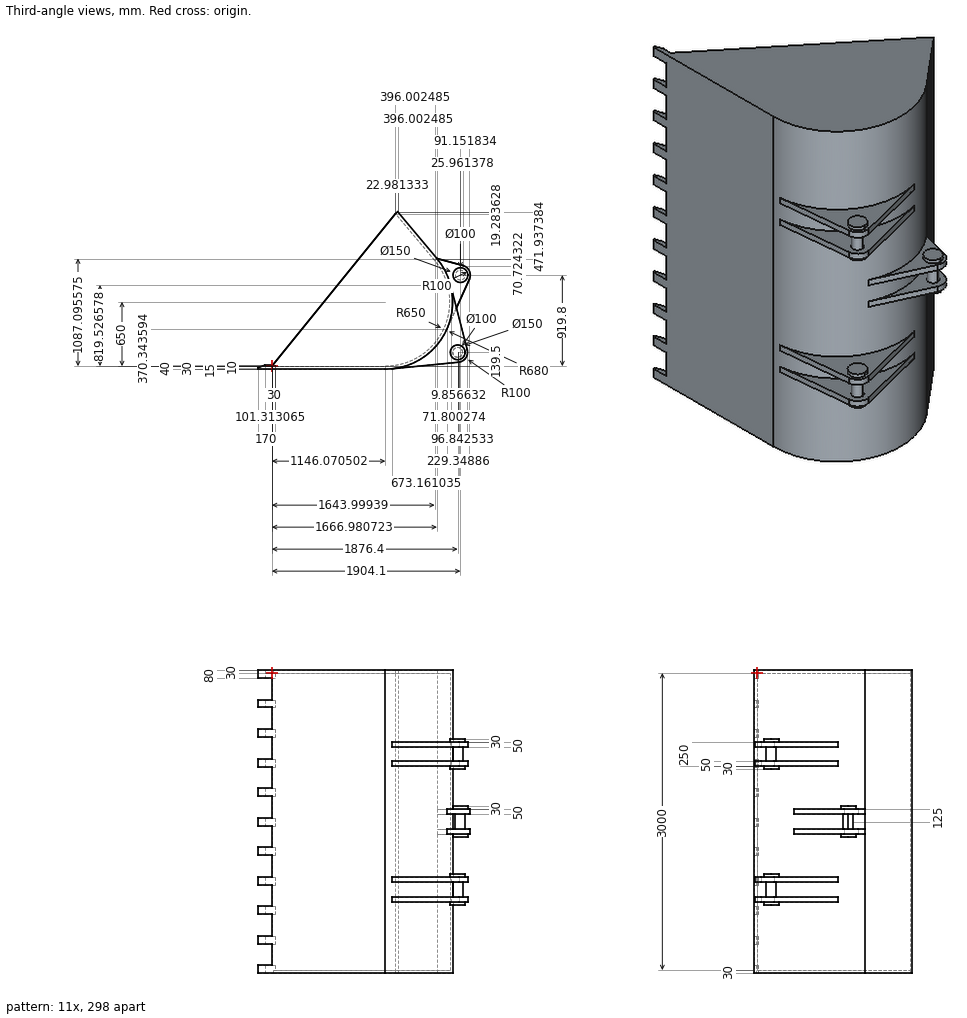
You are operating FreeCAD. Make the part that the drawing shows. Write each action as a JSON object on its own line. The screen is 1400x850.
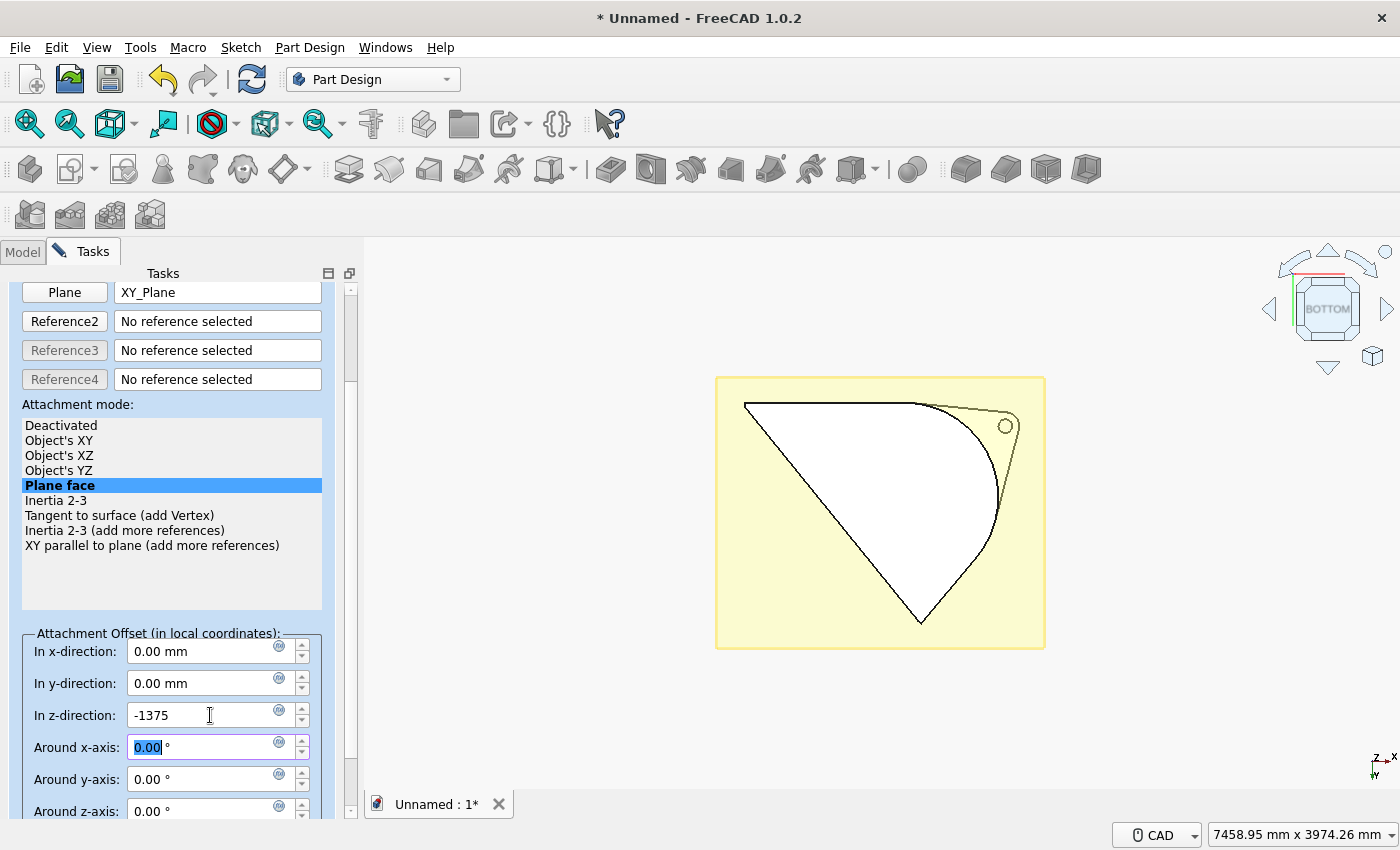
{"action": "scroll", "coordinate": [351, 550], "scroll_direction": "up", "scroll_amount": 3}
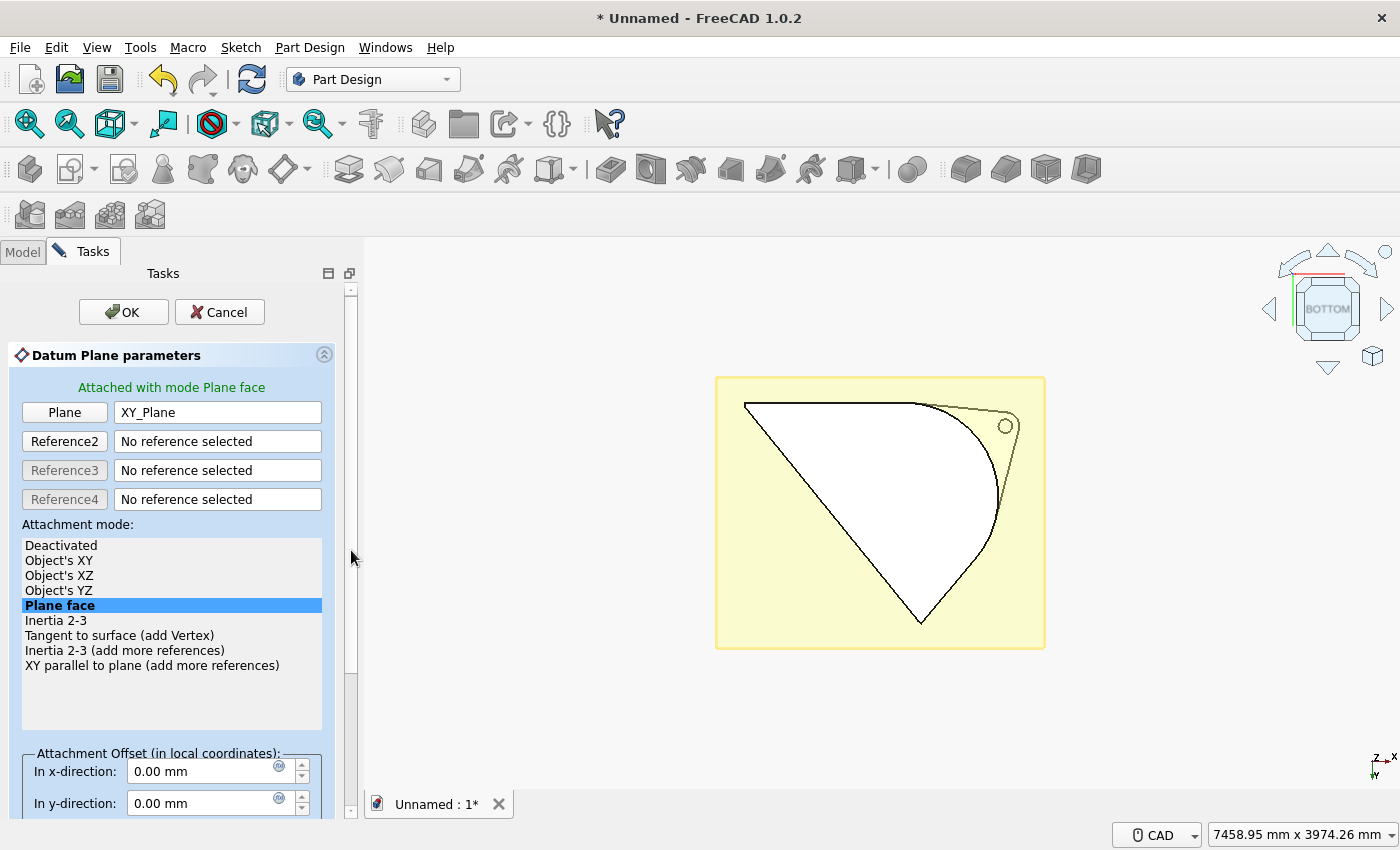
{"action": "left_click", "coordinate": [124, 312]}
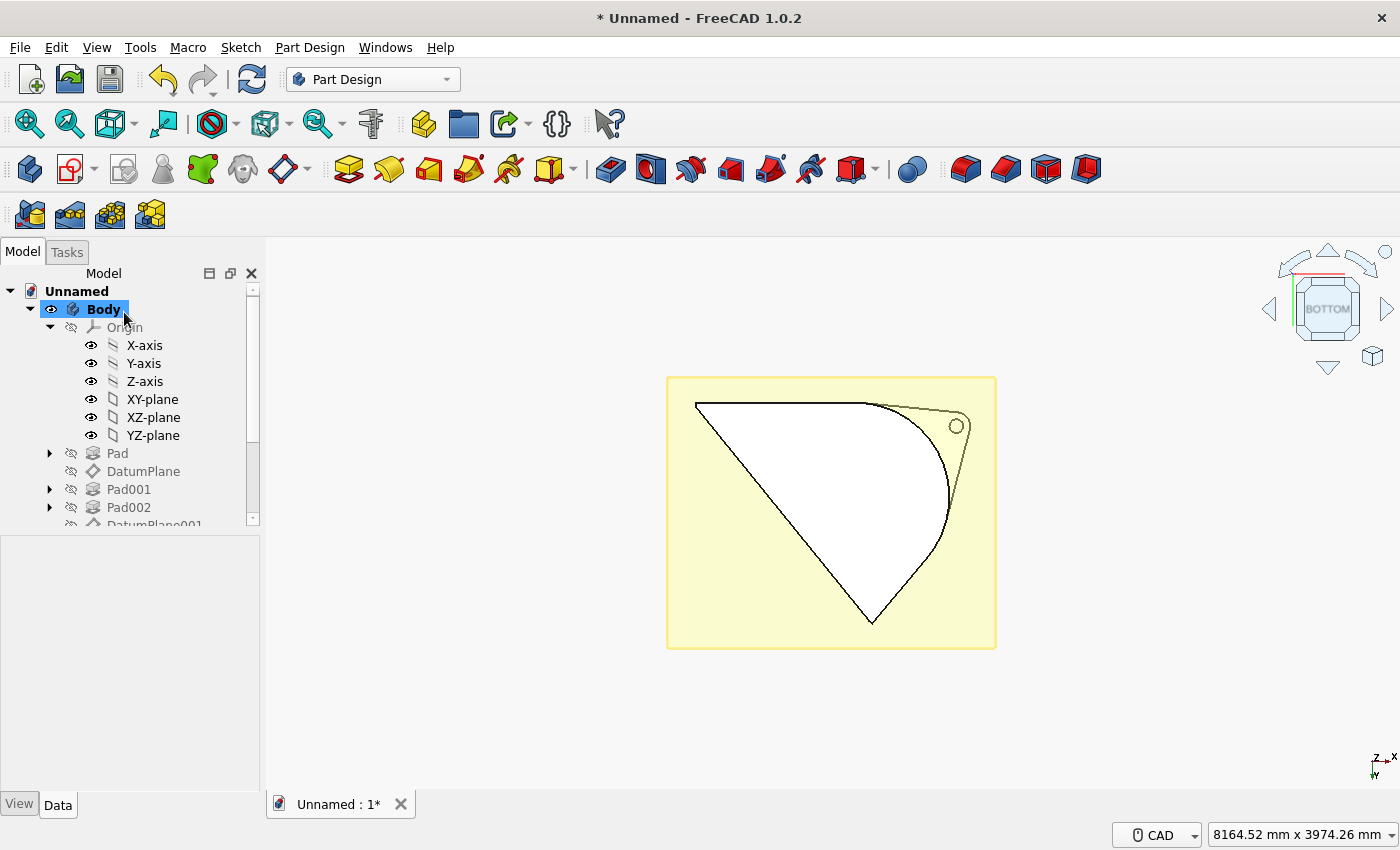
{"action": "scroll", "coordinate": [100, 413], "scroll_direction": "down", "scroll_amount": 3}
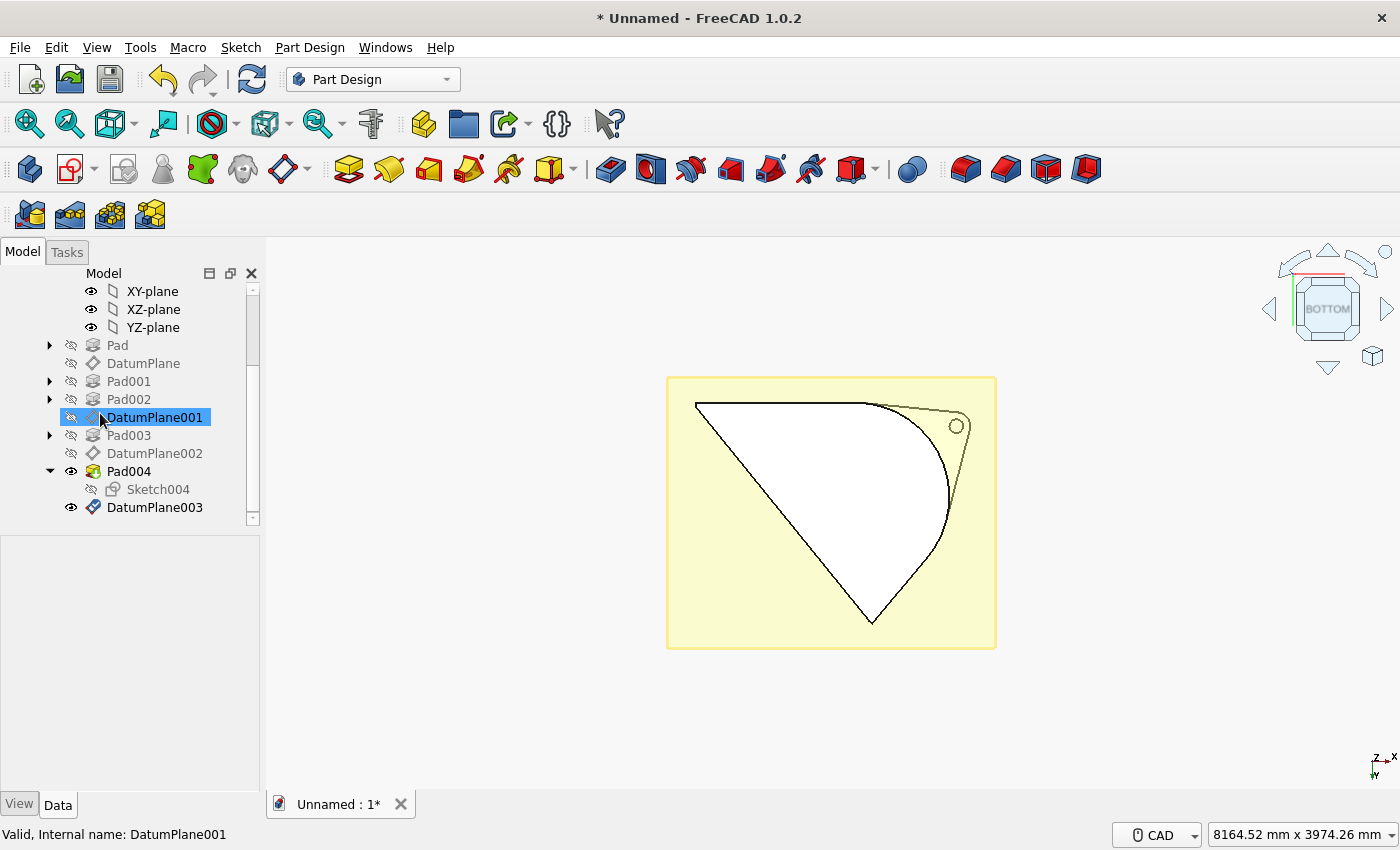
{"action": "left_click", "coordinate": [116, 507]}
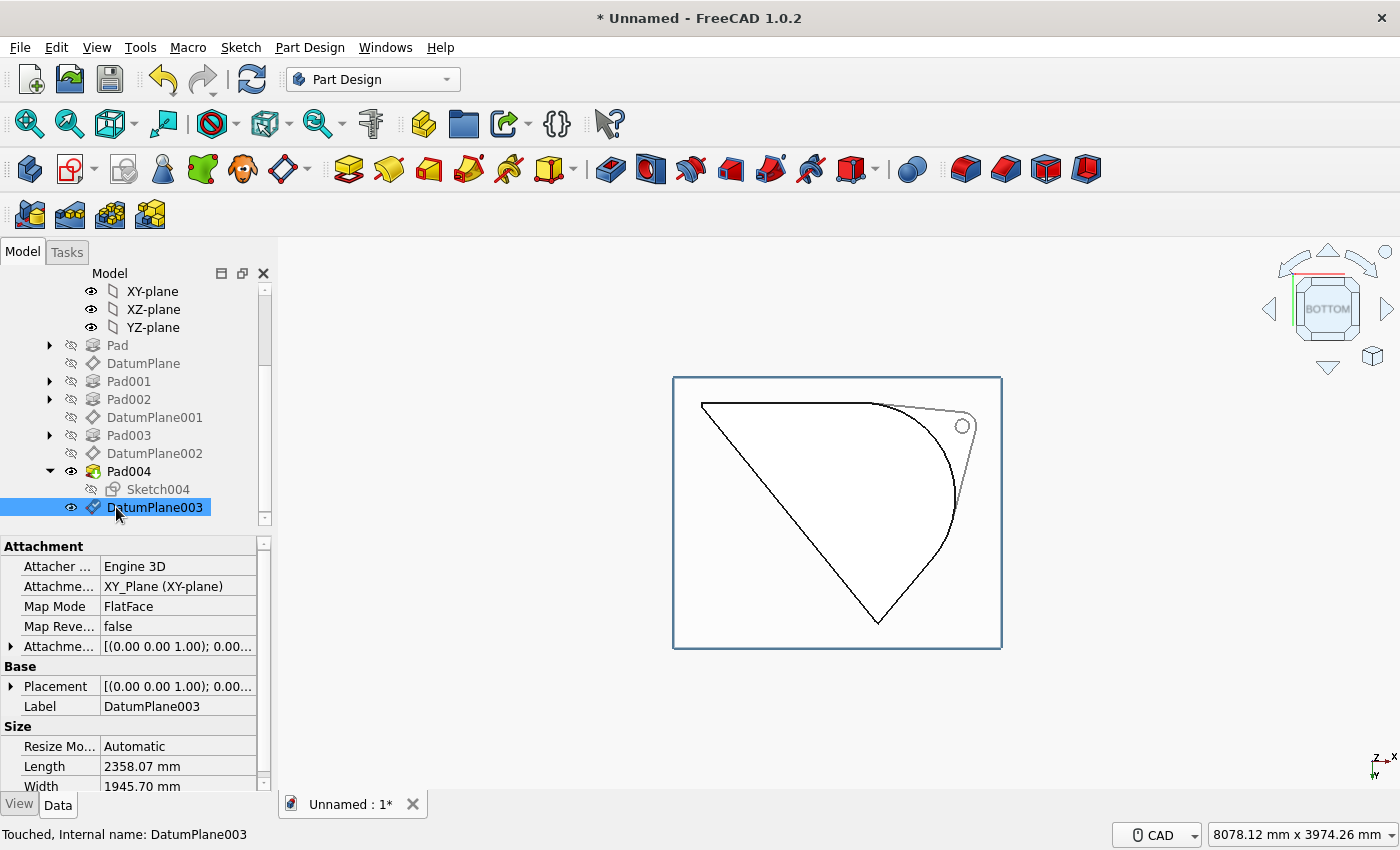
{"action": "left_click", "coordinate": [70, 170]}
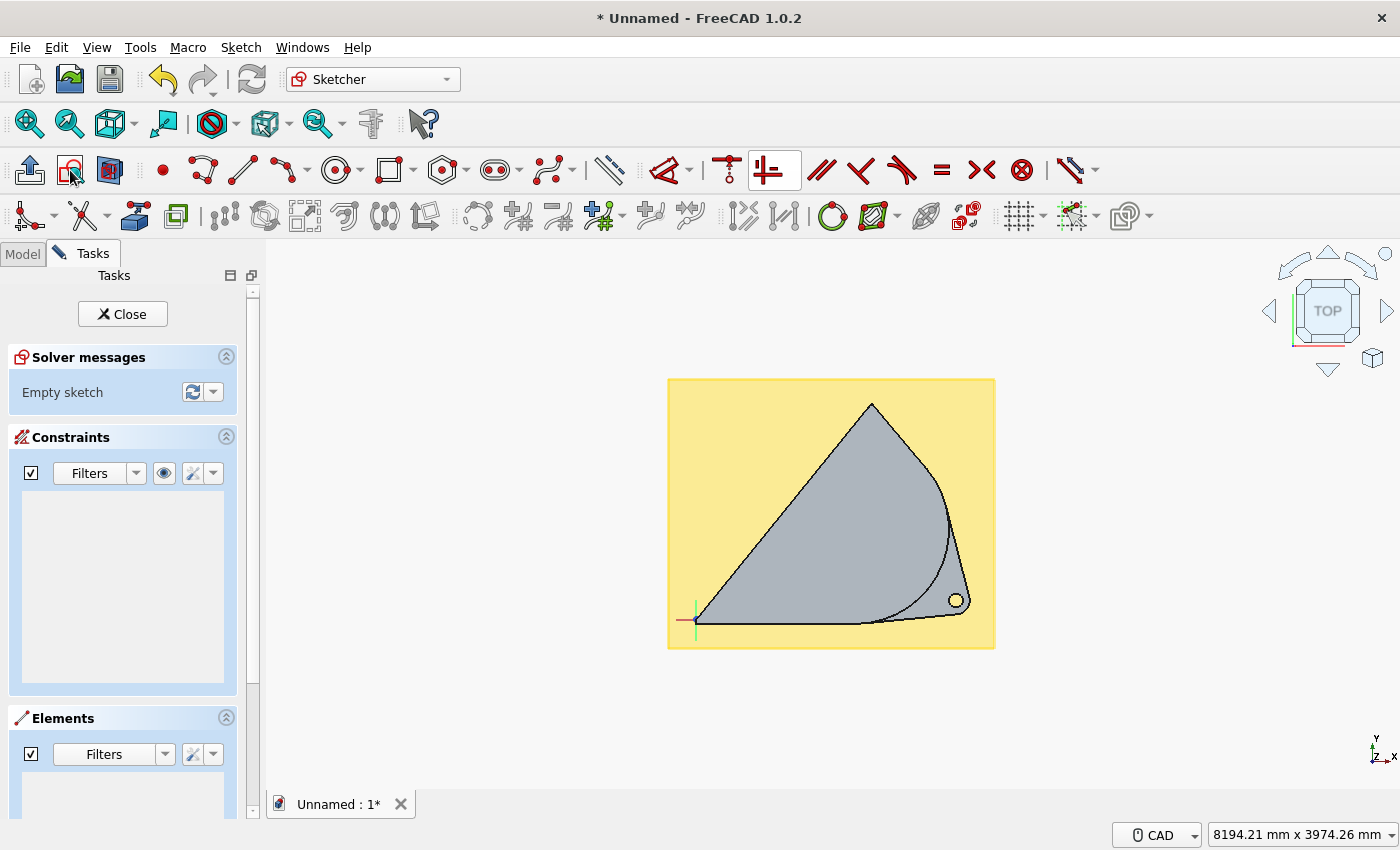
{"action": "left_click", "coordinate": [110, 170]}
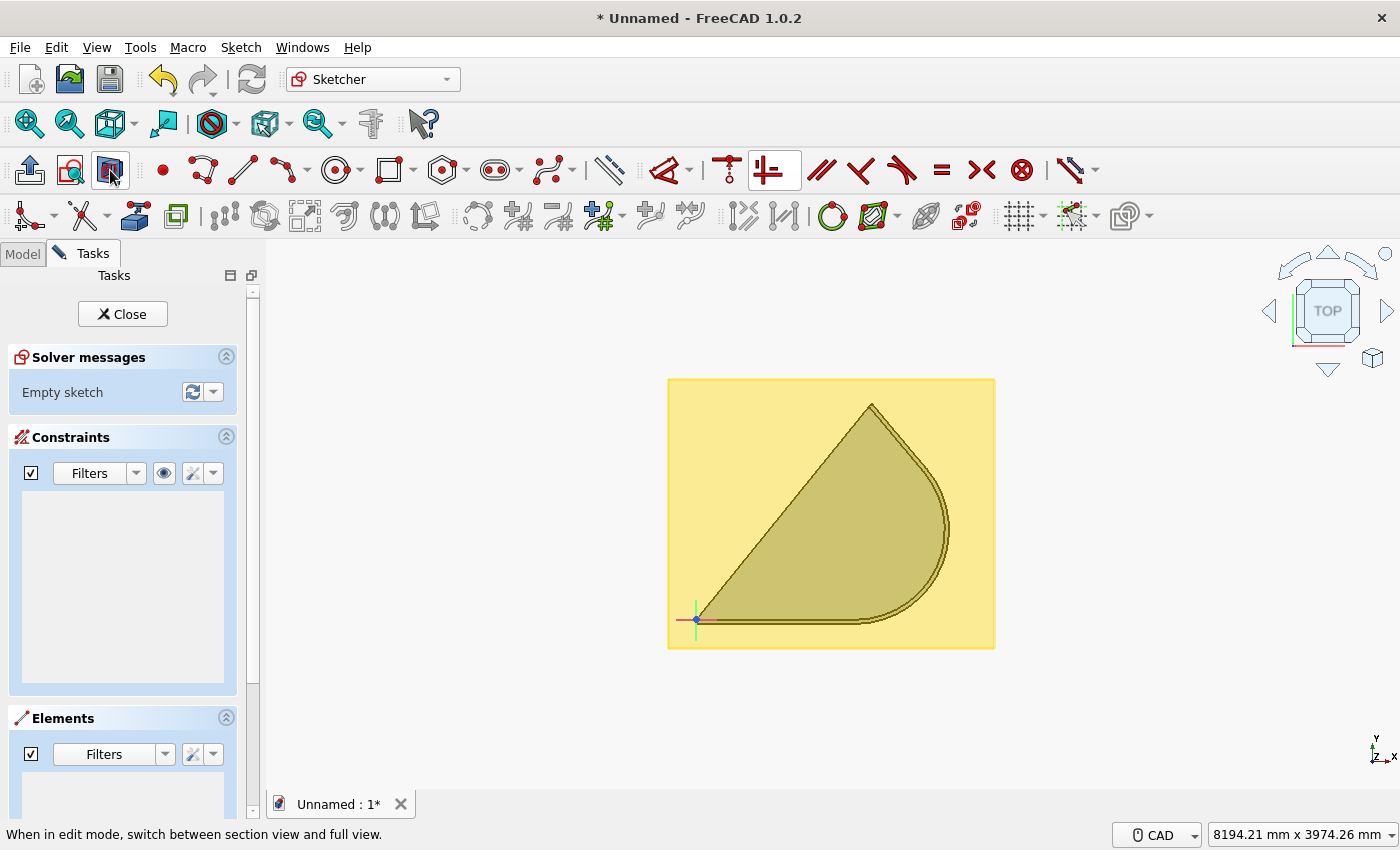
{"action": "scroll", "coordinate": [1029, 521], "scroll_direction": "up", "scroll_amount": 6}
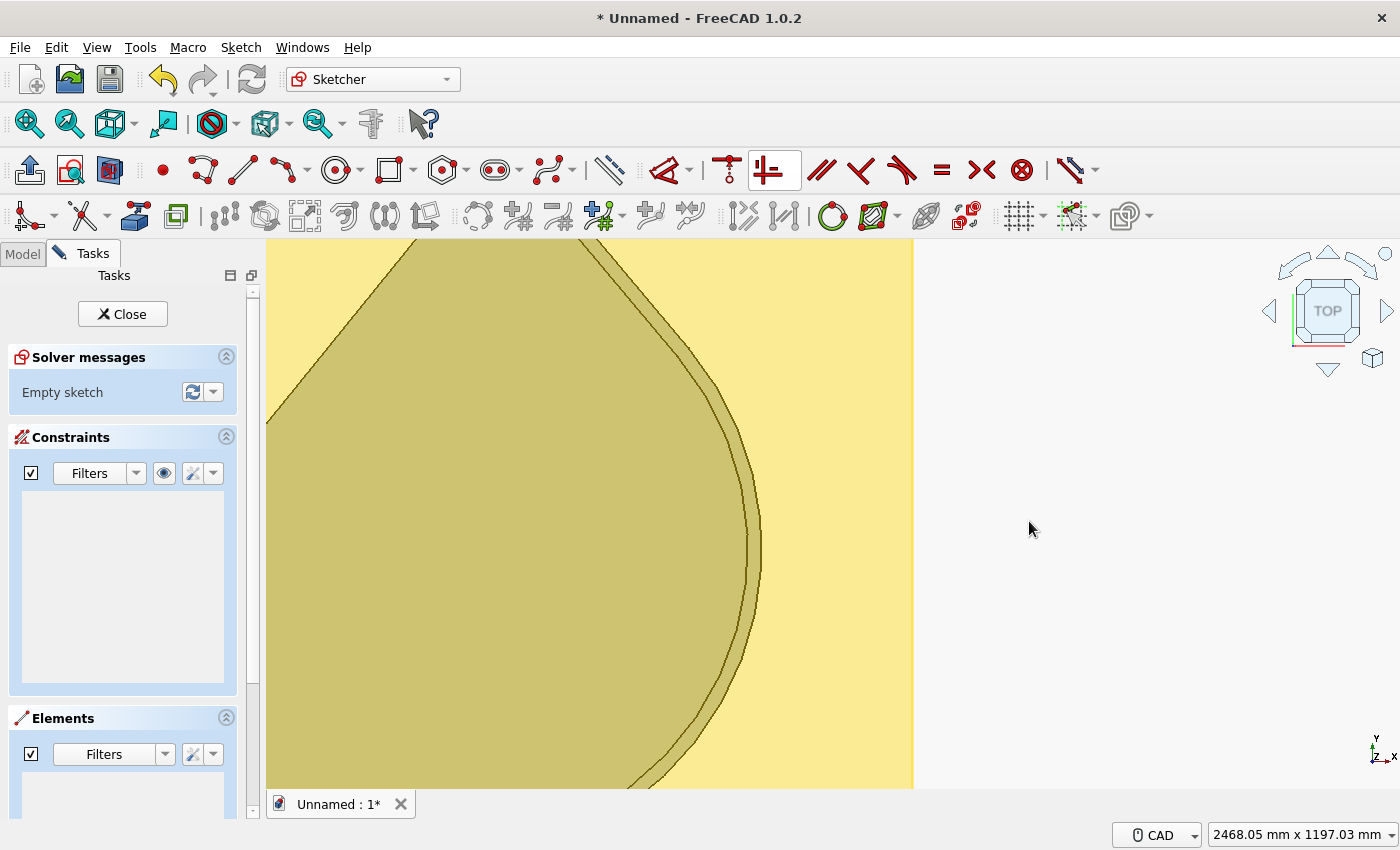
{"action": "key", "text": "g l"}